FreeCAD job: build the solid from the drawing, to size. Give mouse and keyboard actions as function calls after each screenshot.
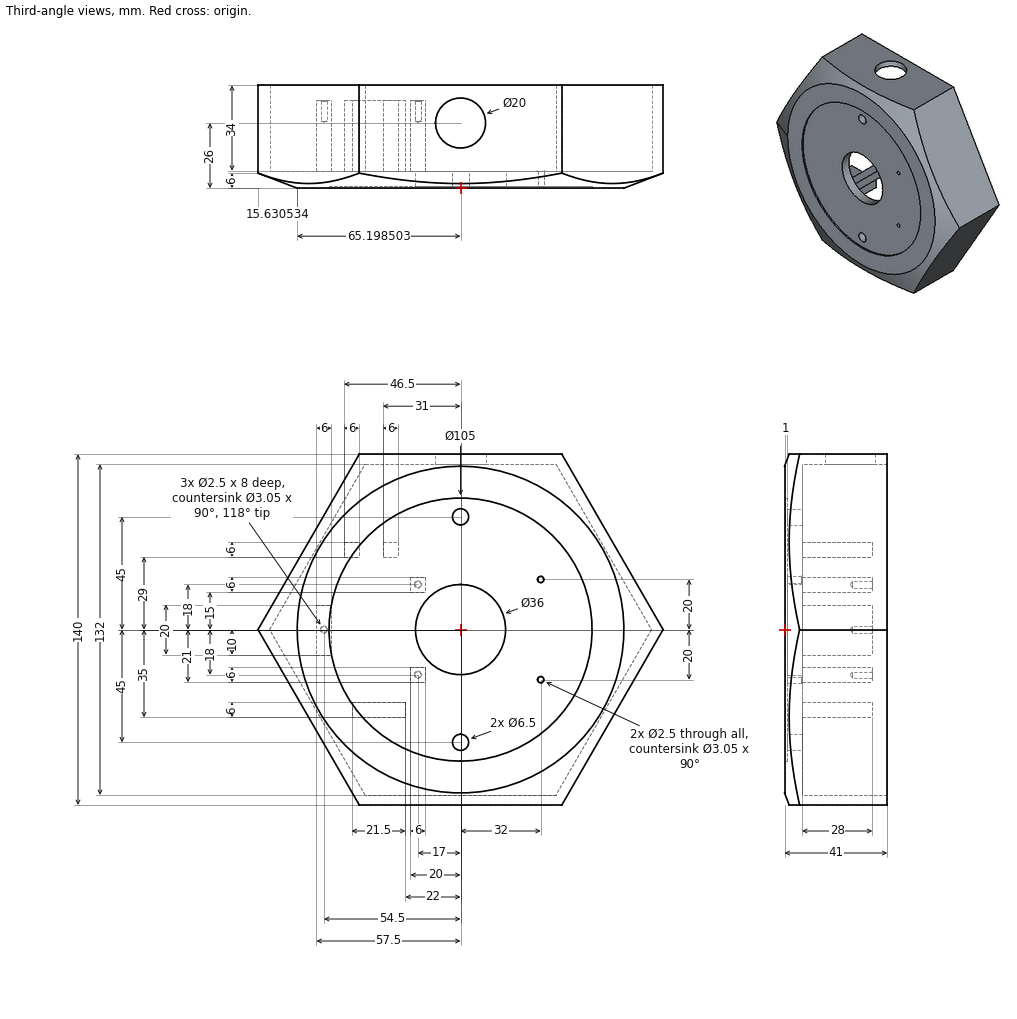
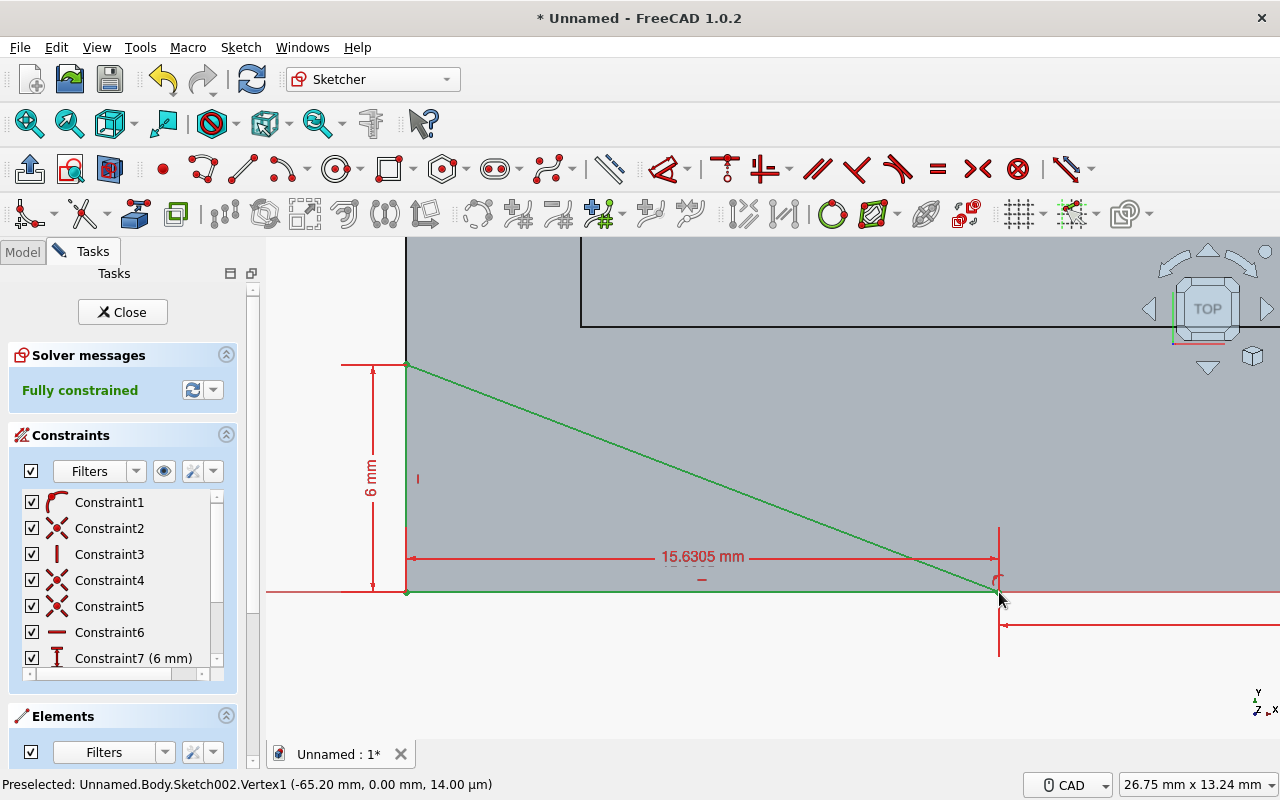
click(123, 312)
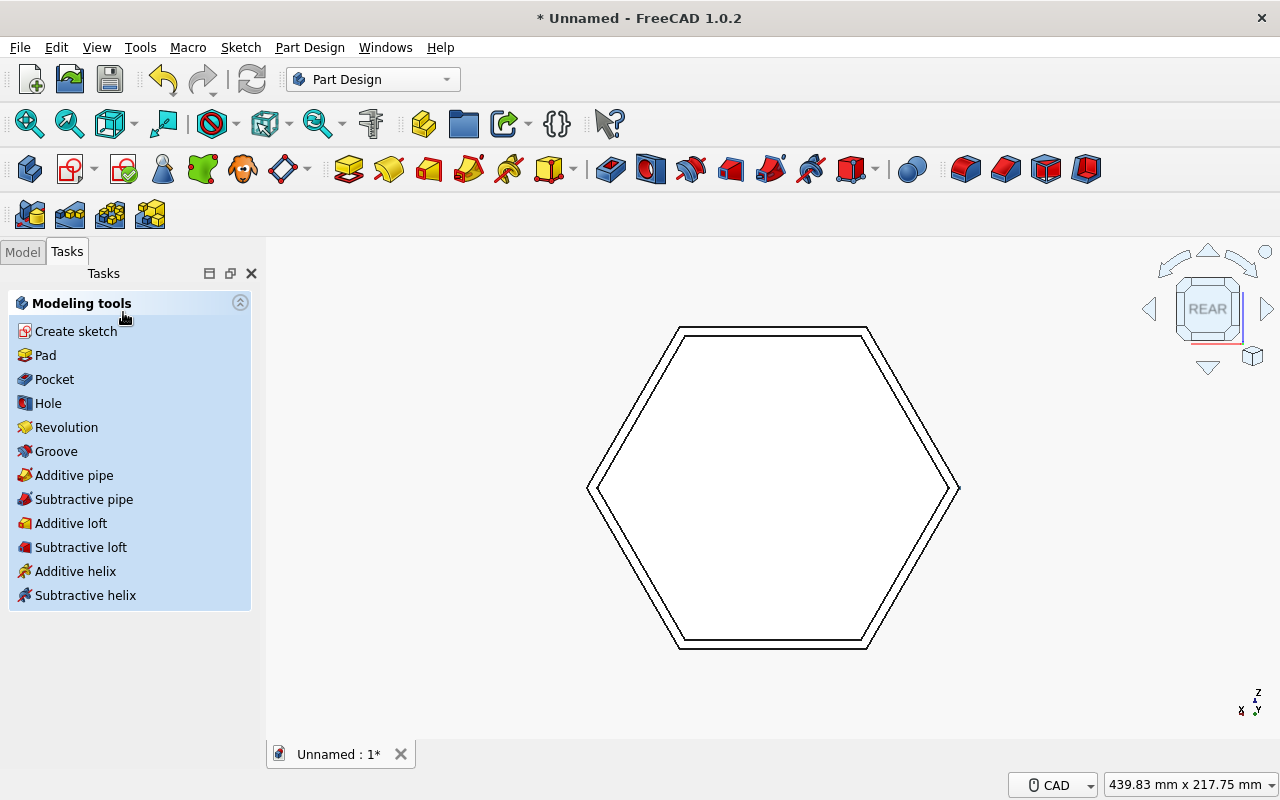
click(692, 170)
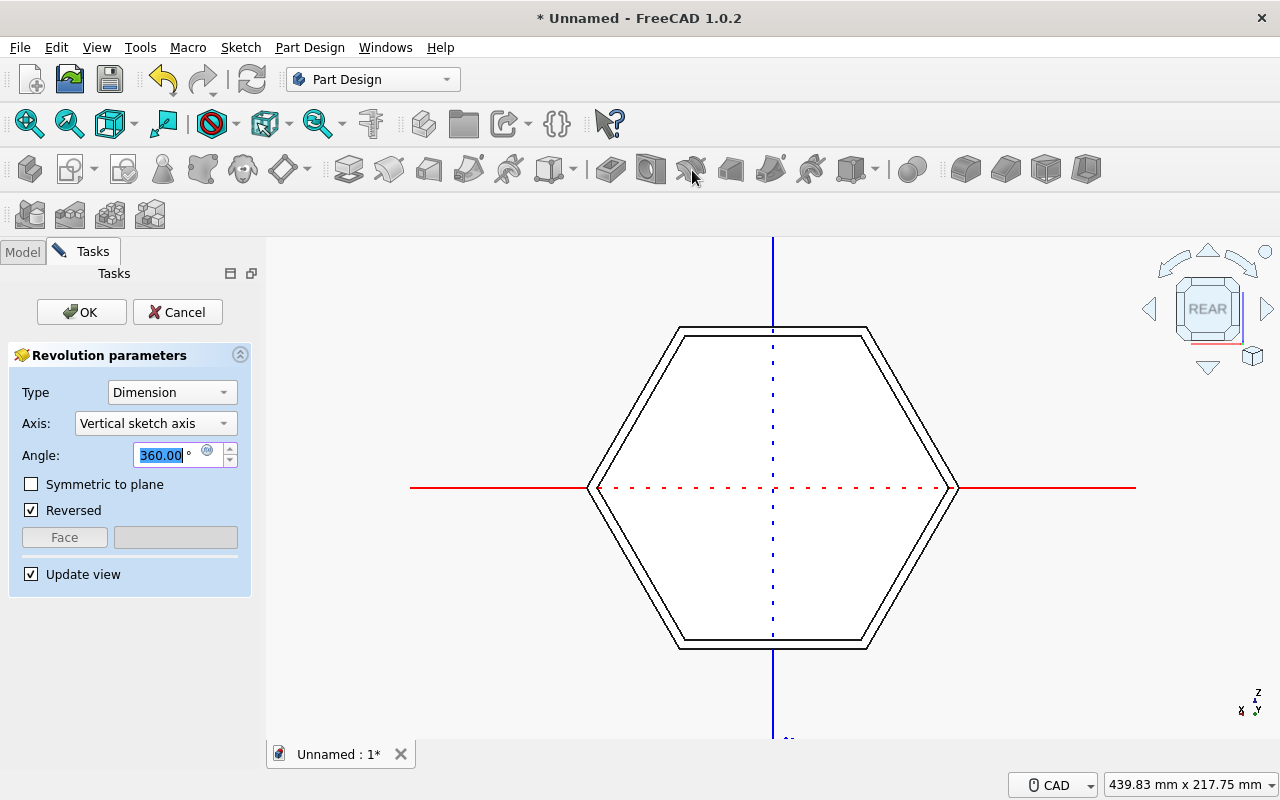
click(82, 312)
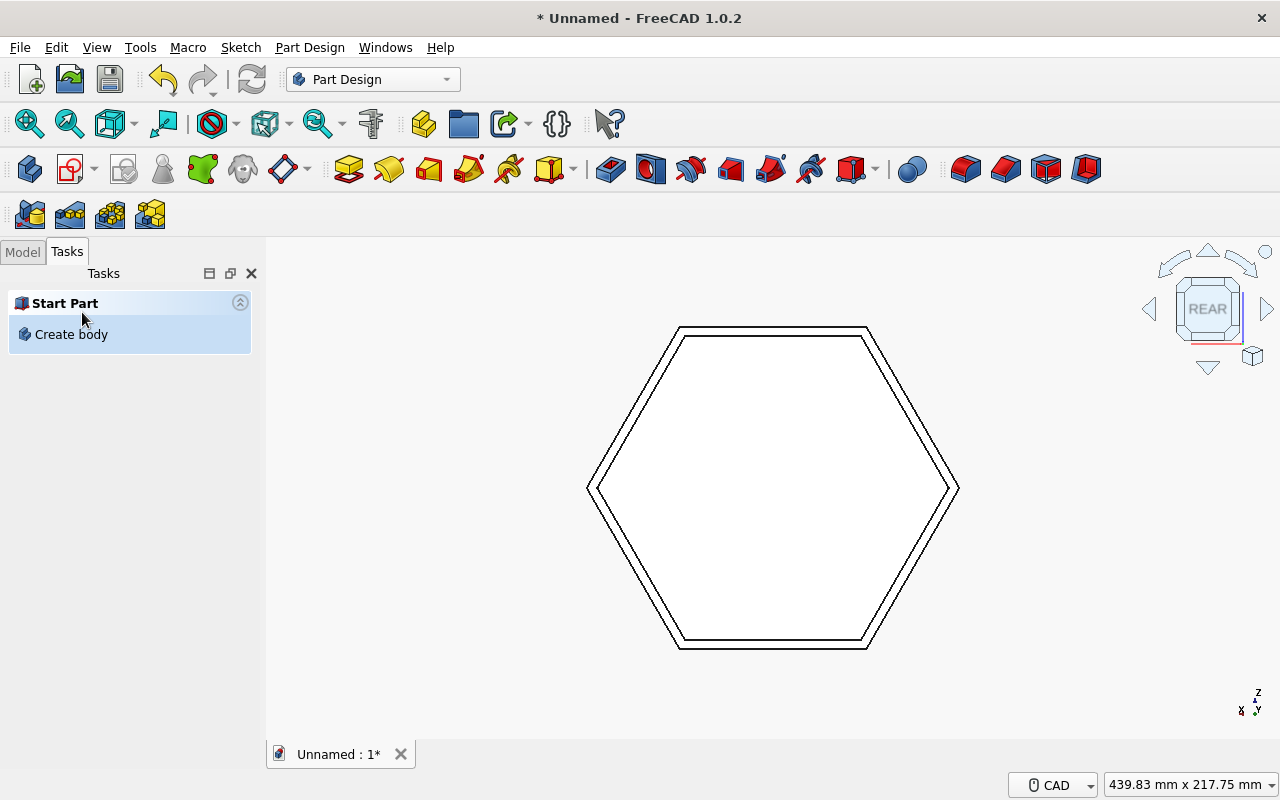
click(70, 170)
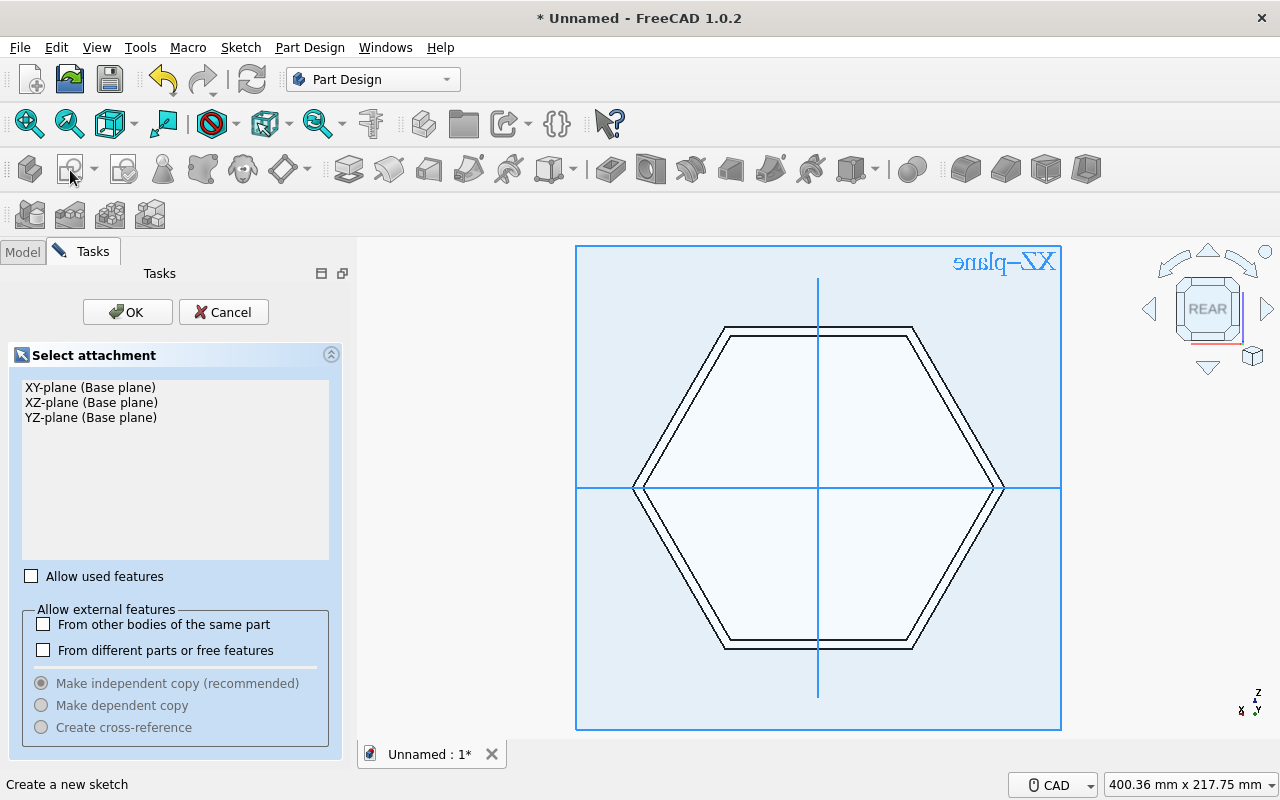
click(82, 402)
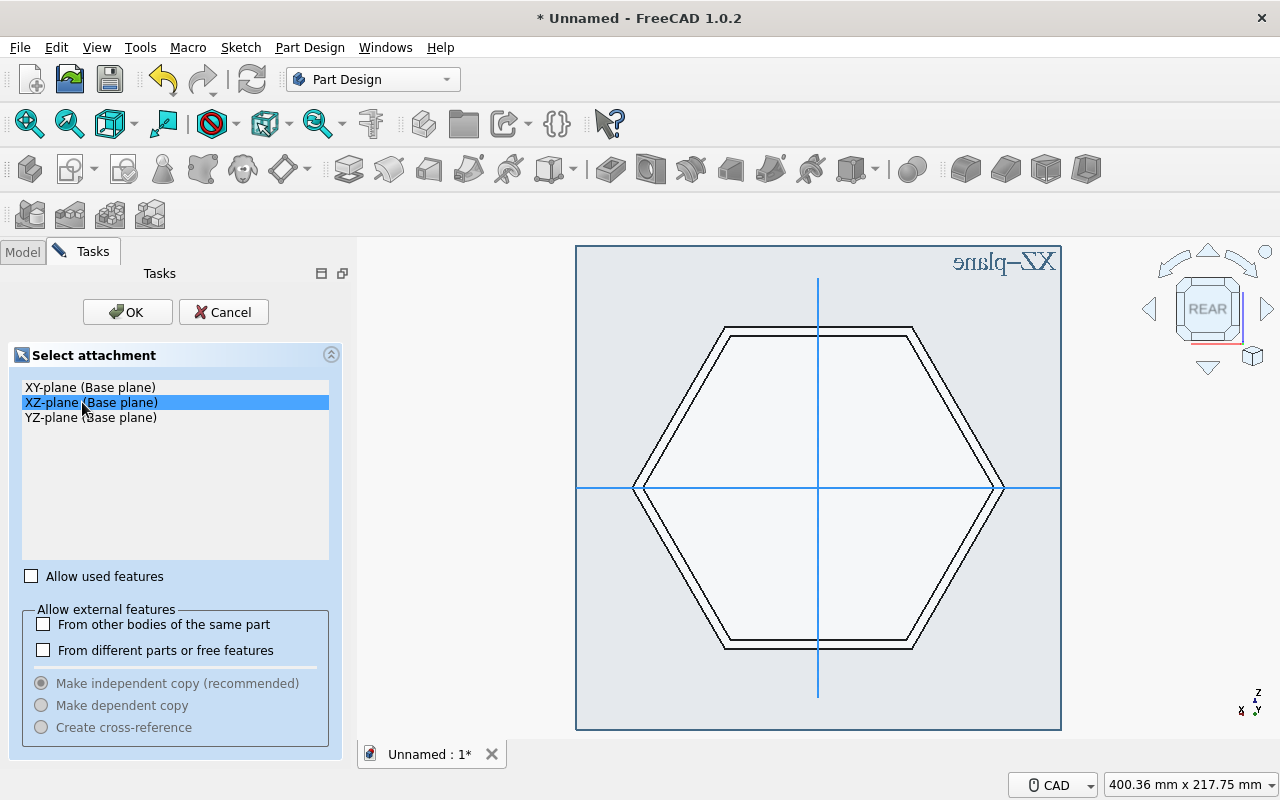
click(128, 312)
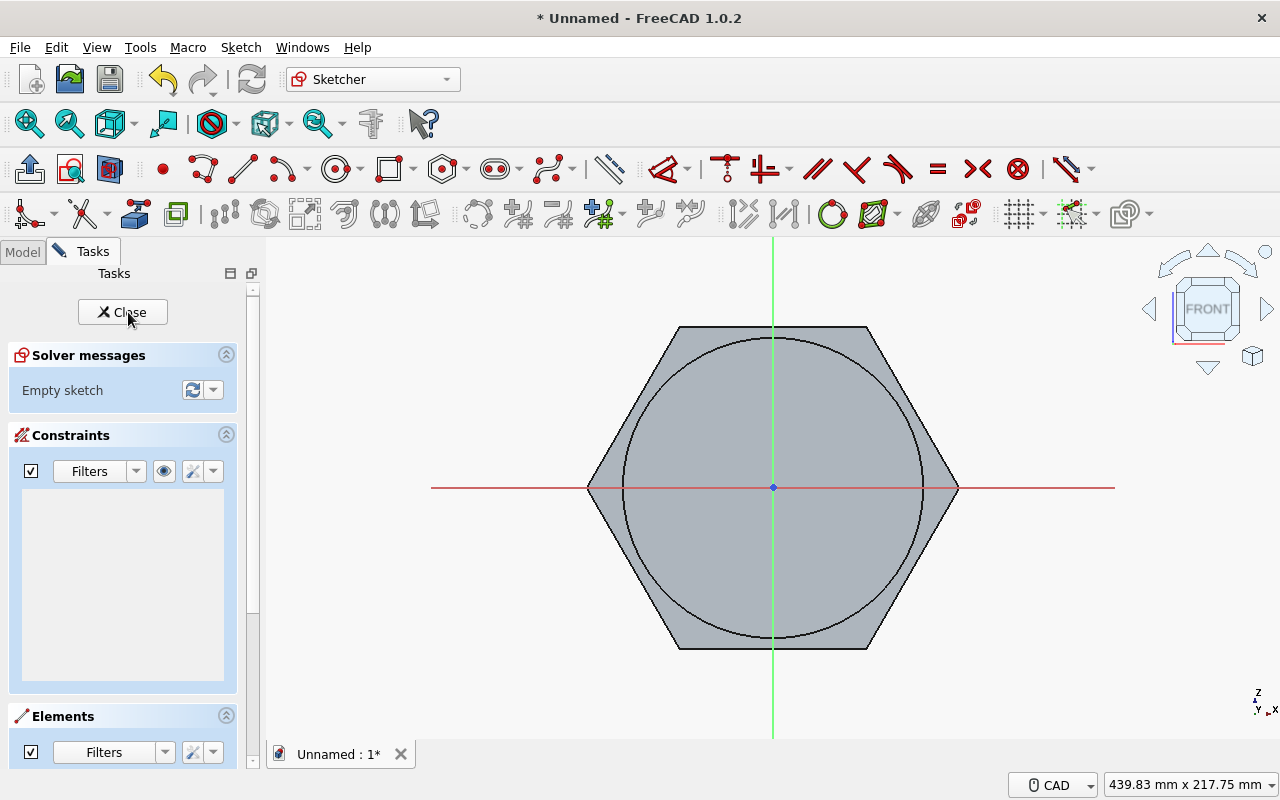
key(g)
key(c)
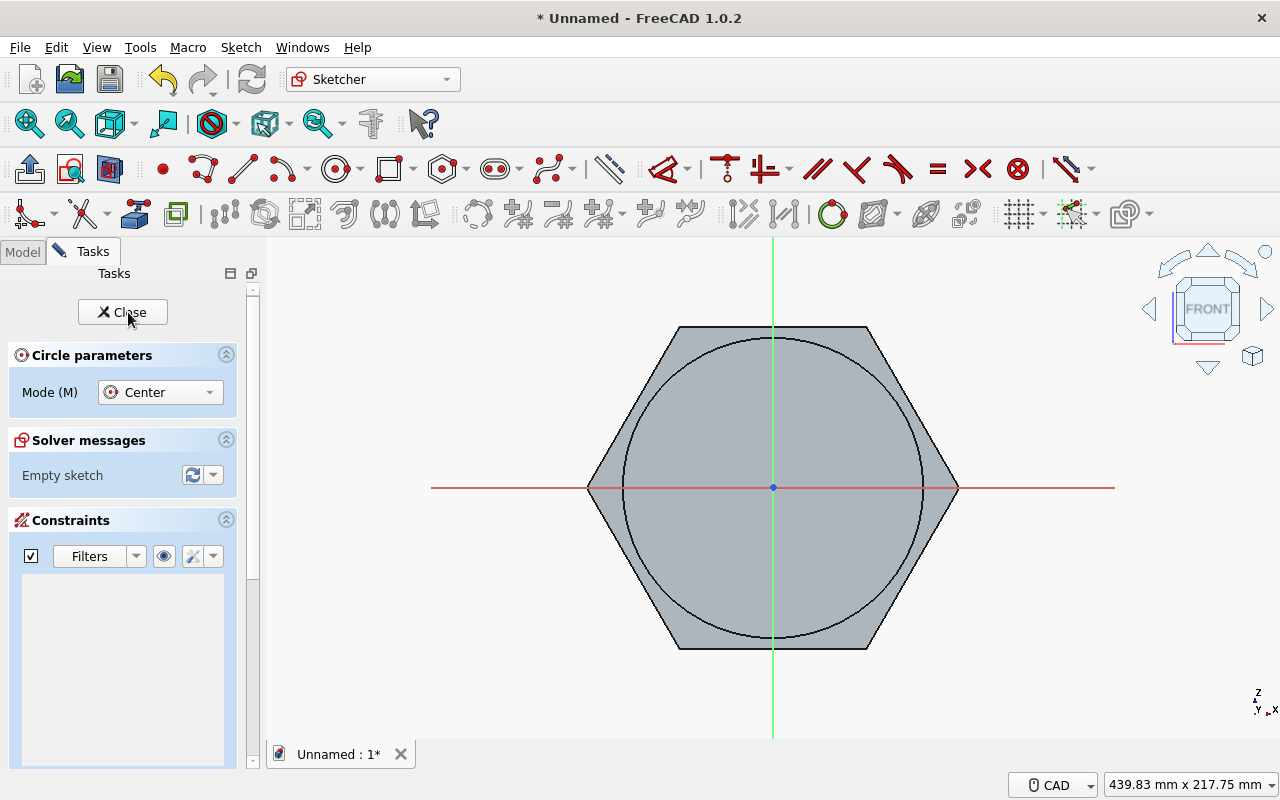
click(773, 488)
move(859, 402)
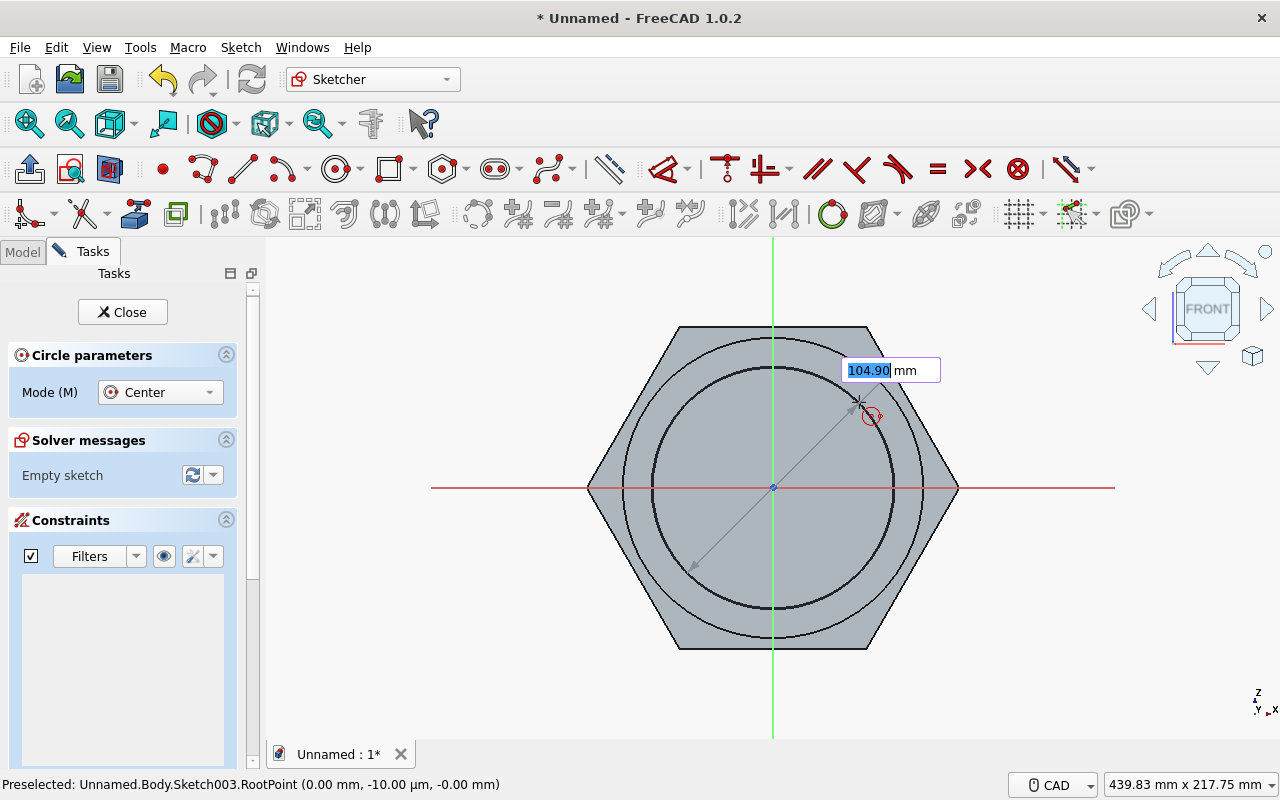
text(105)
key(Return)
key(Escape)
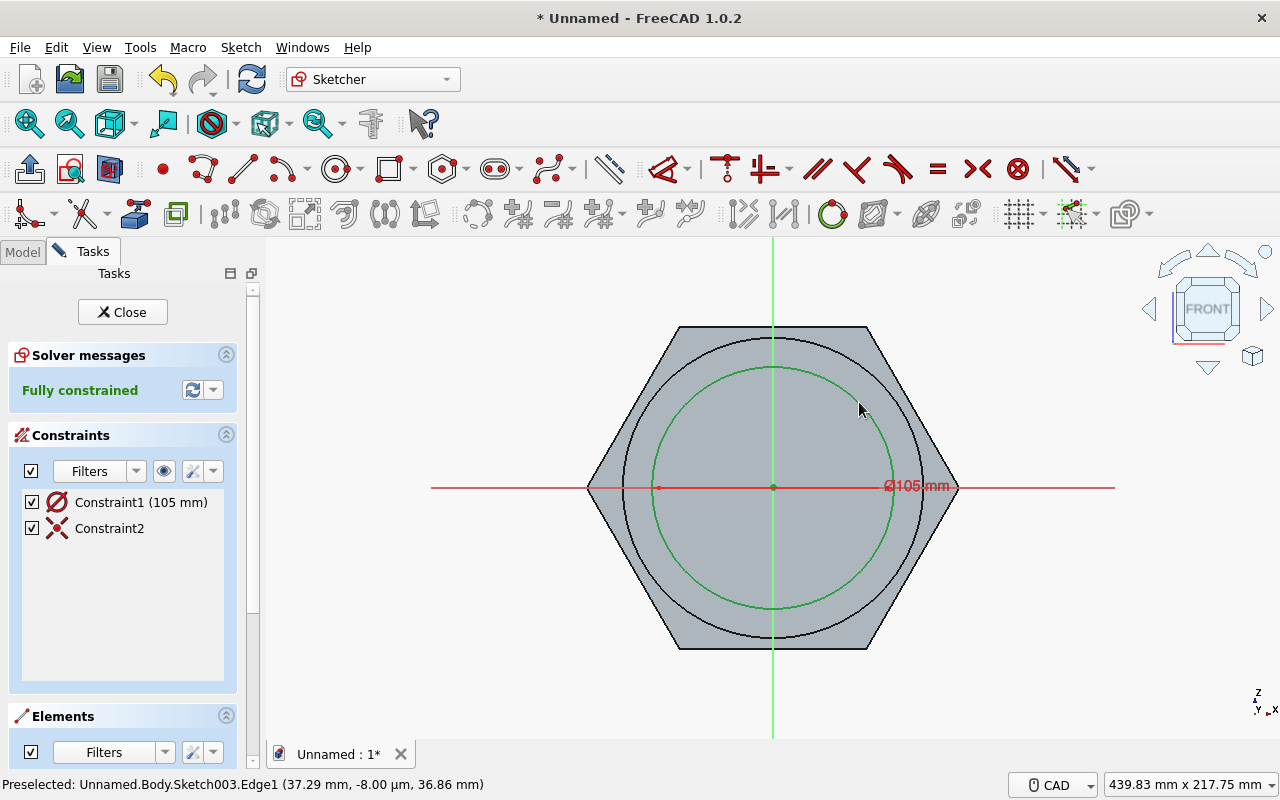
click(123, 312)